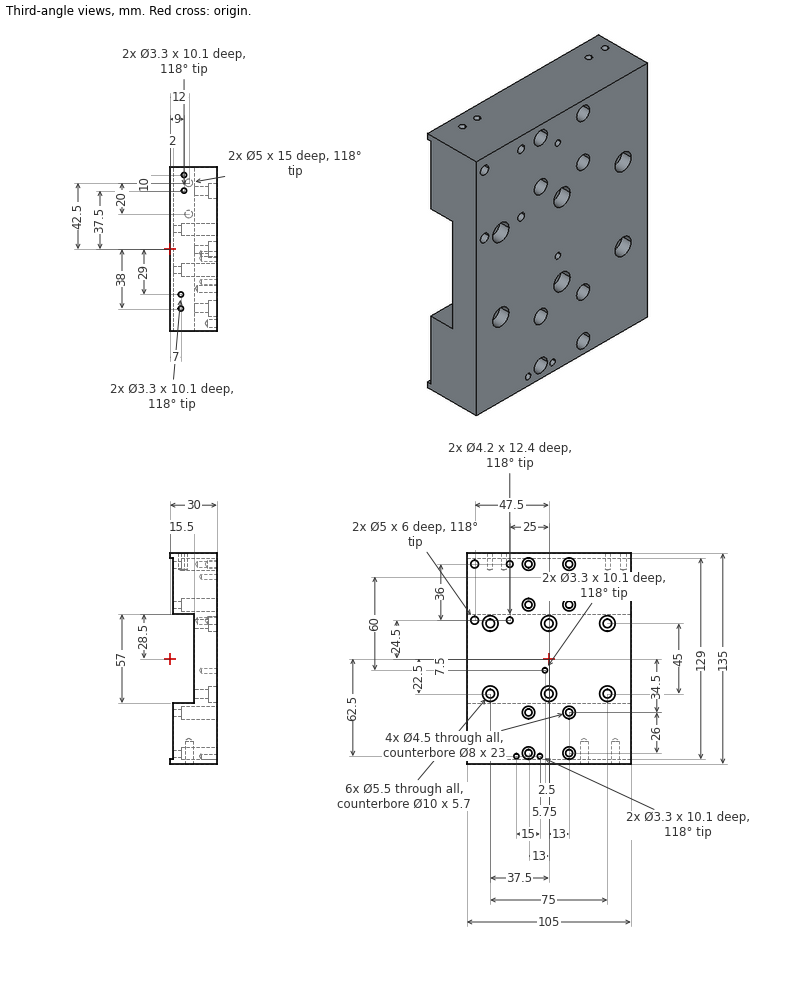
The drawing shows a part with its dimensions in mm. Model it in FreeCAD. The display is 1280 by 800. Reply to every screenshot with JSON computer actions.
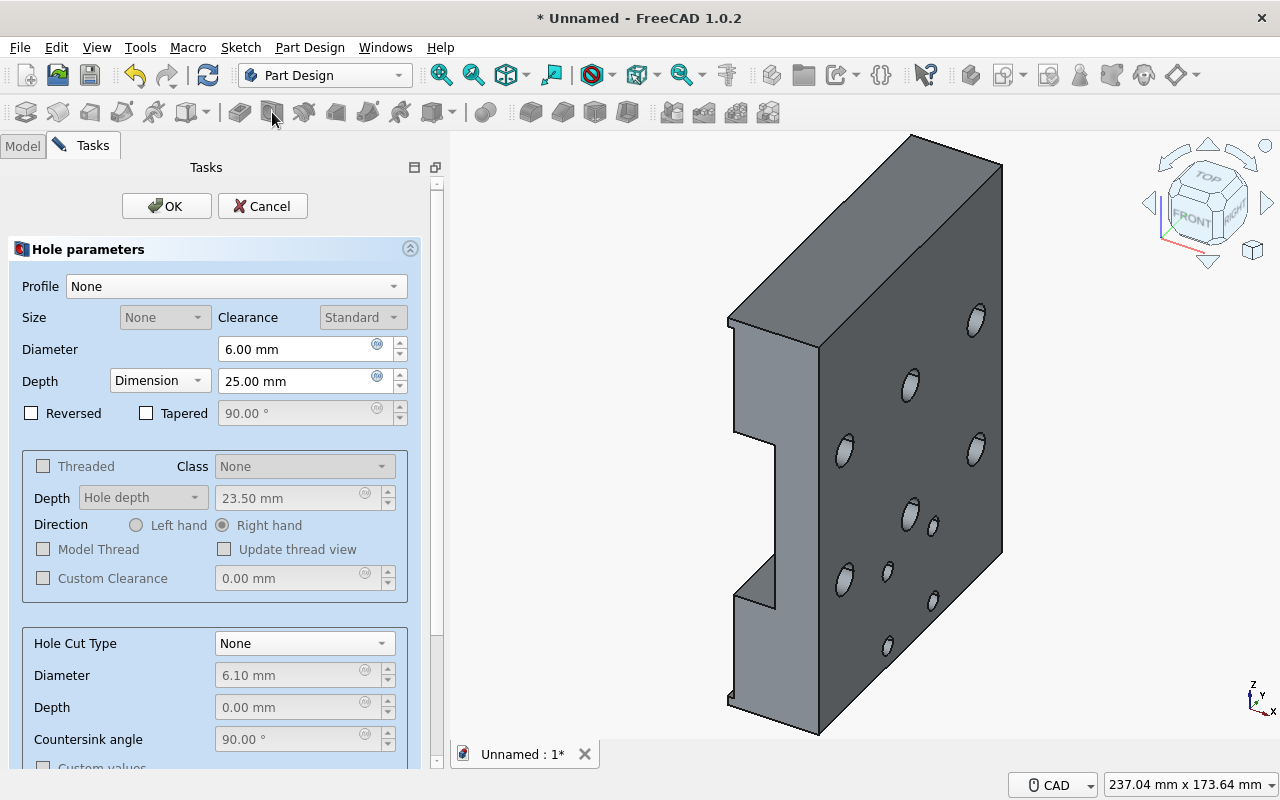
{"action": "triple_click", "coordinate": [305, 349]}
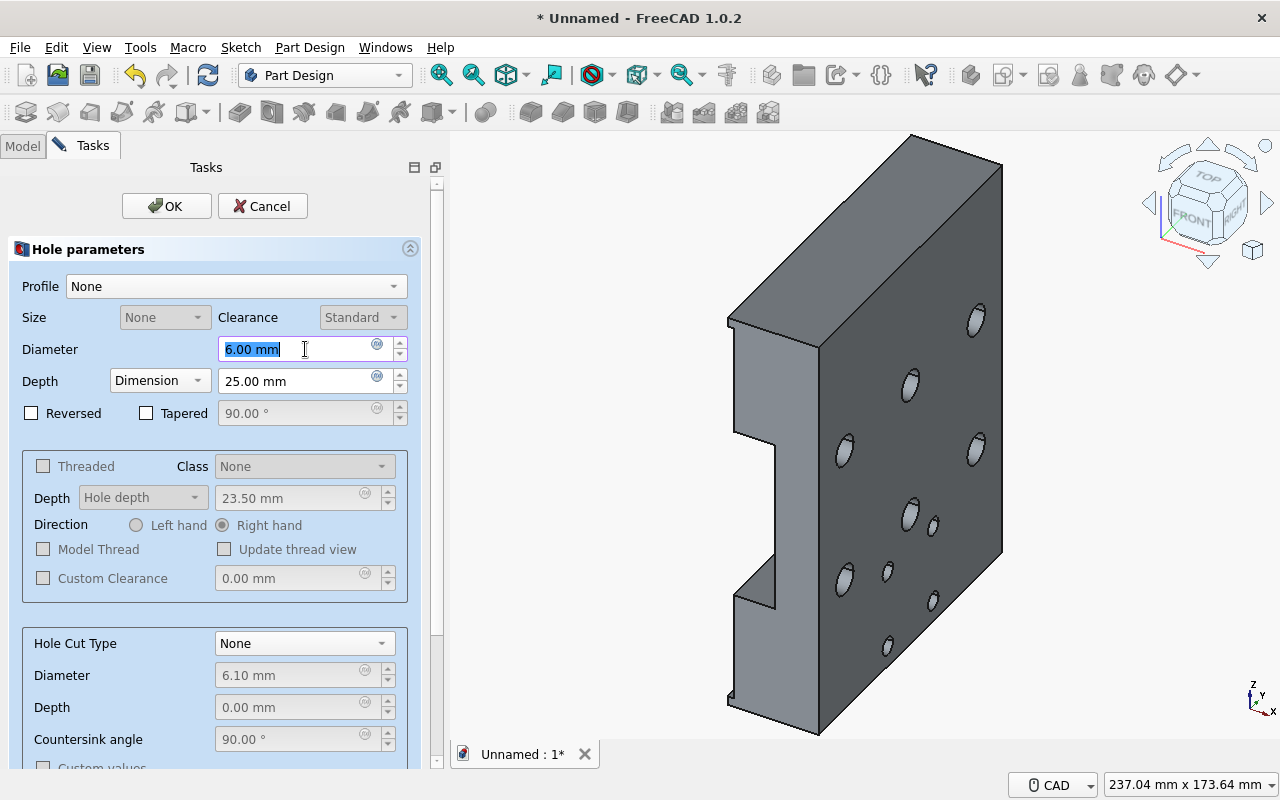
{"action": "type", "text": "4.5"}
{"action": "key", "text": "Tab"}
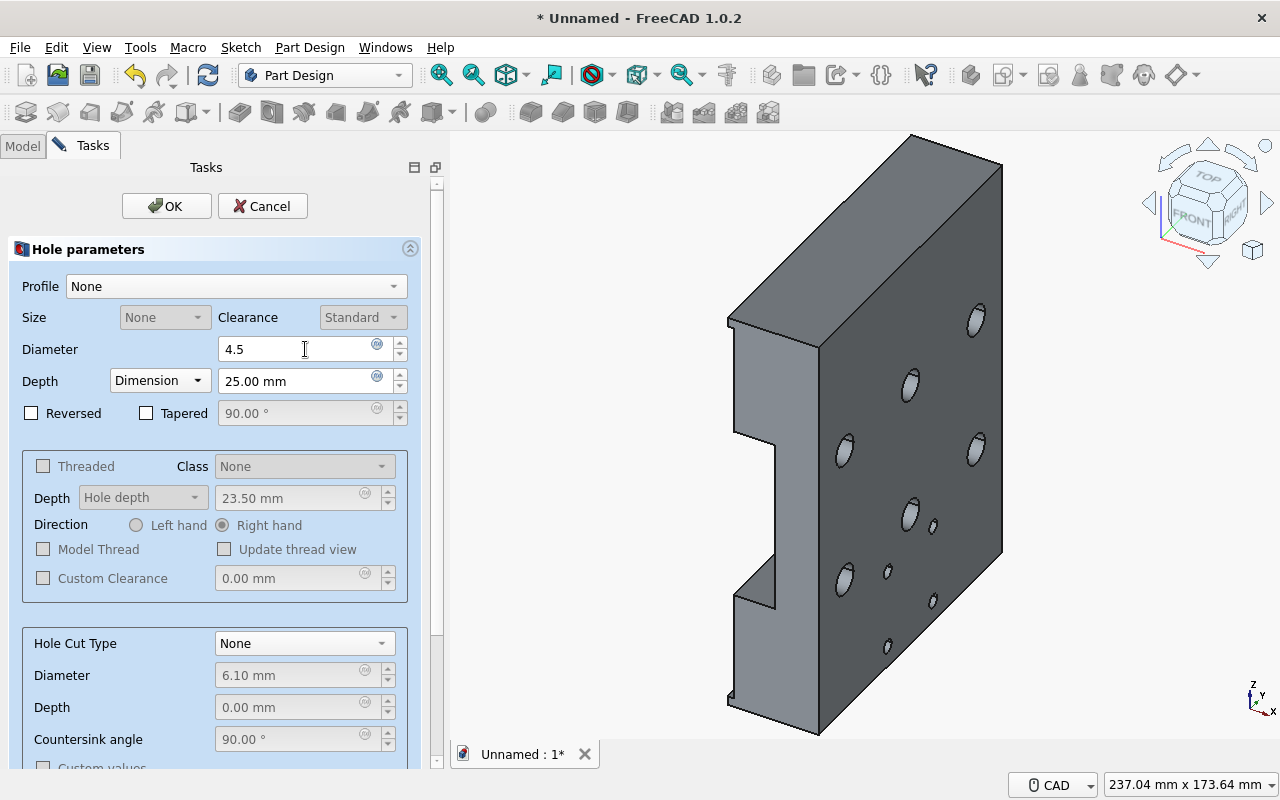
{"action": "left_click", "coordinate": [161, 380]}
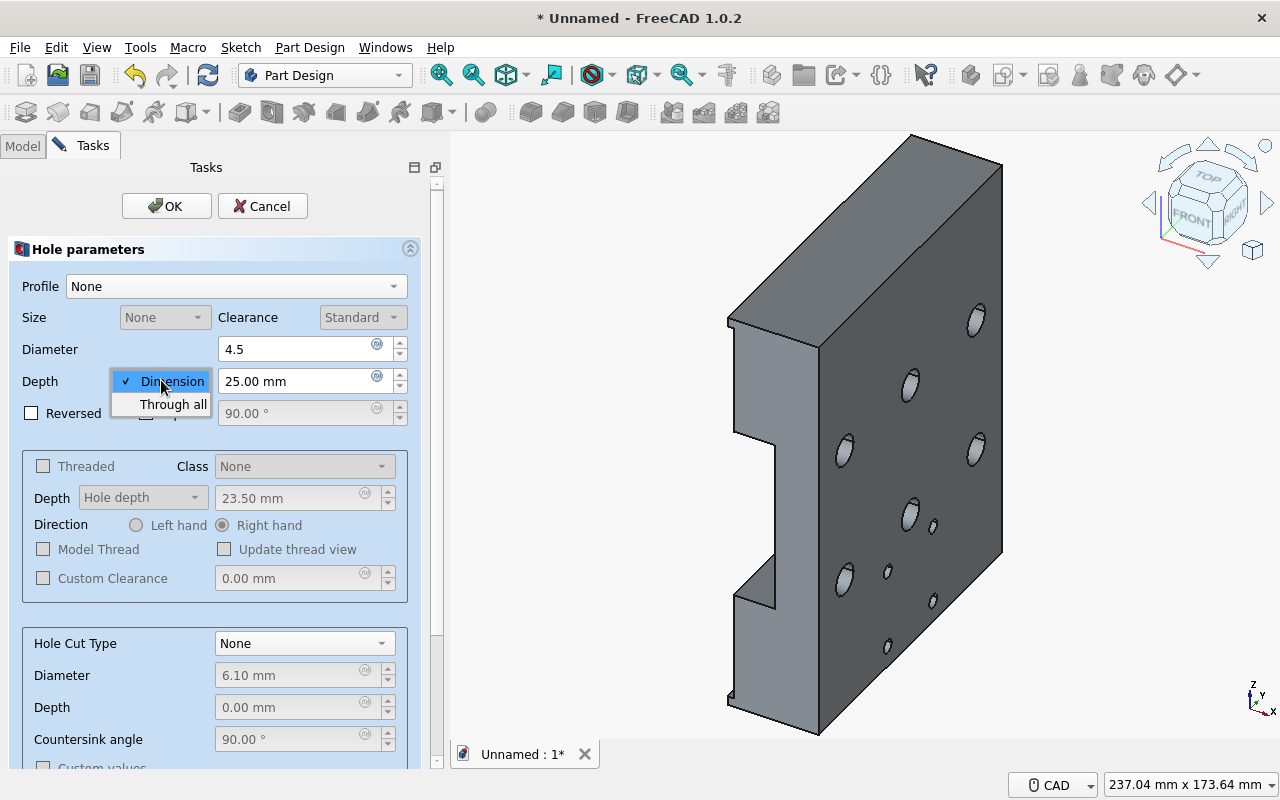
{"action": "left_click", "coordinate": [160, 404]}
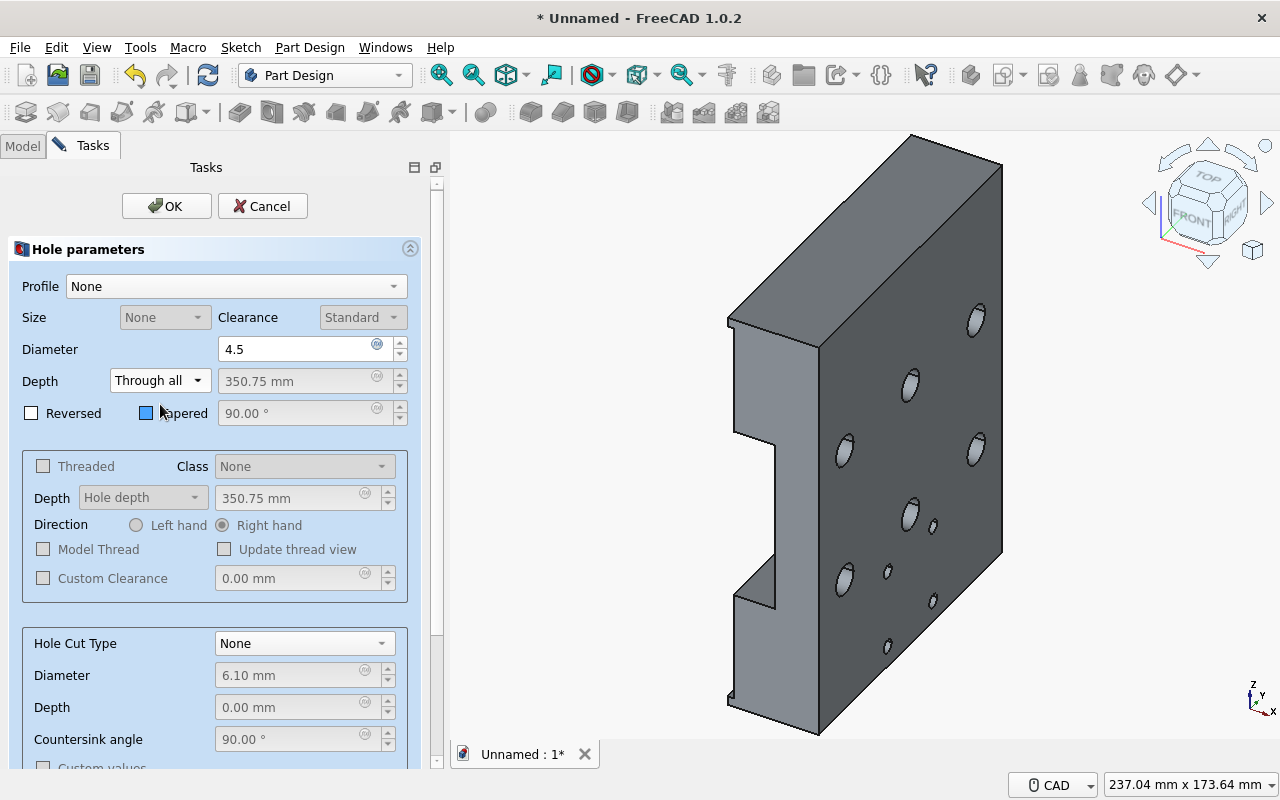
{"action": "left_click", "coordinate": [306, 644]}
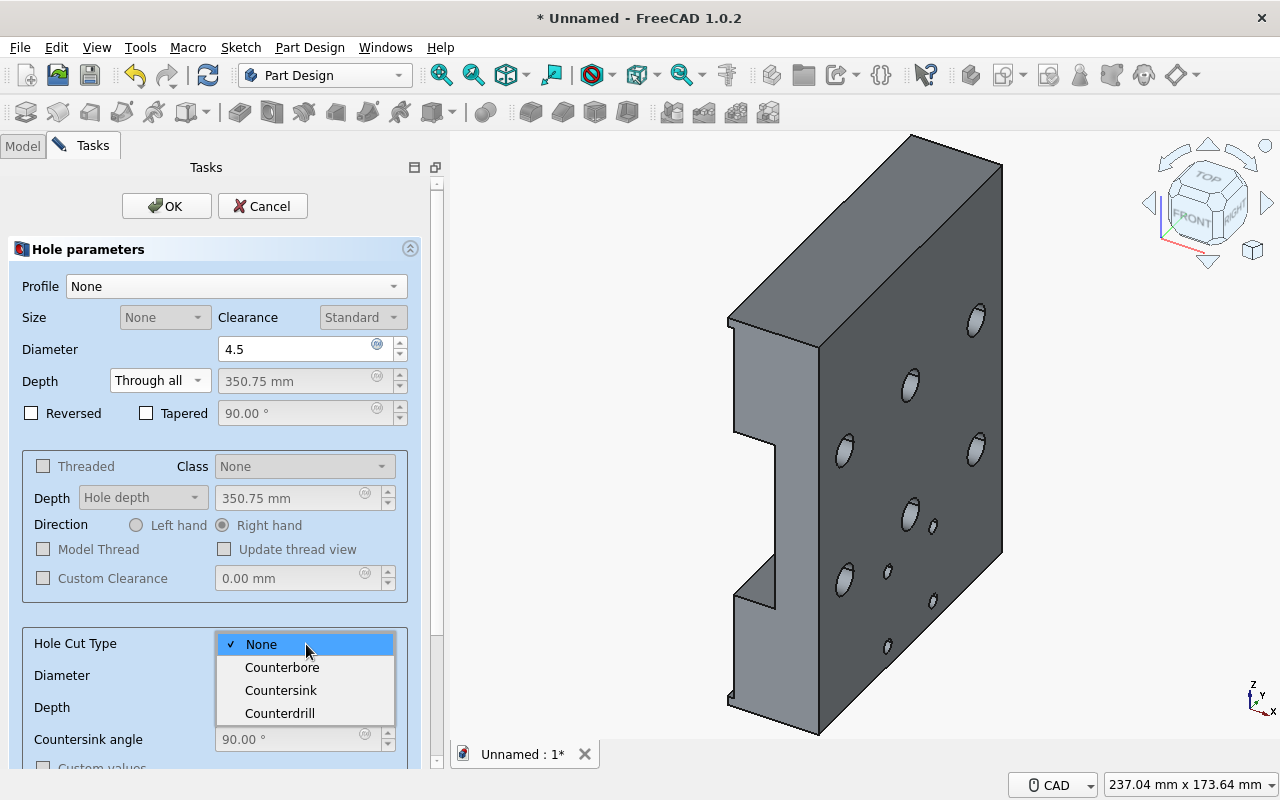
{"action": "left_click", "coordinate": [304, 668]}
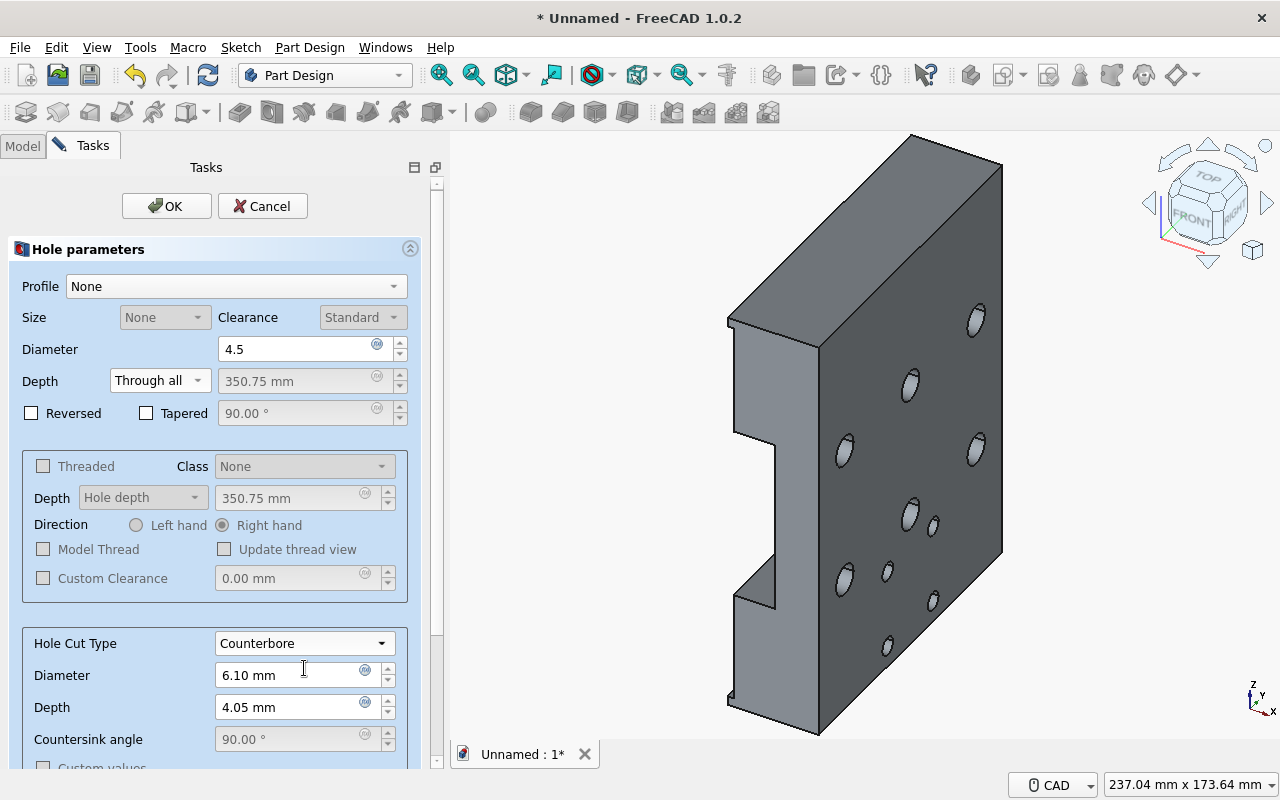
{"action": "triple_click", "coordinate": [298, 675]}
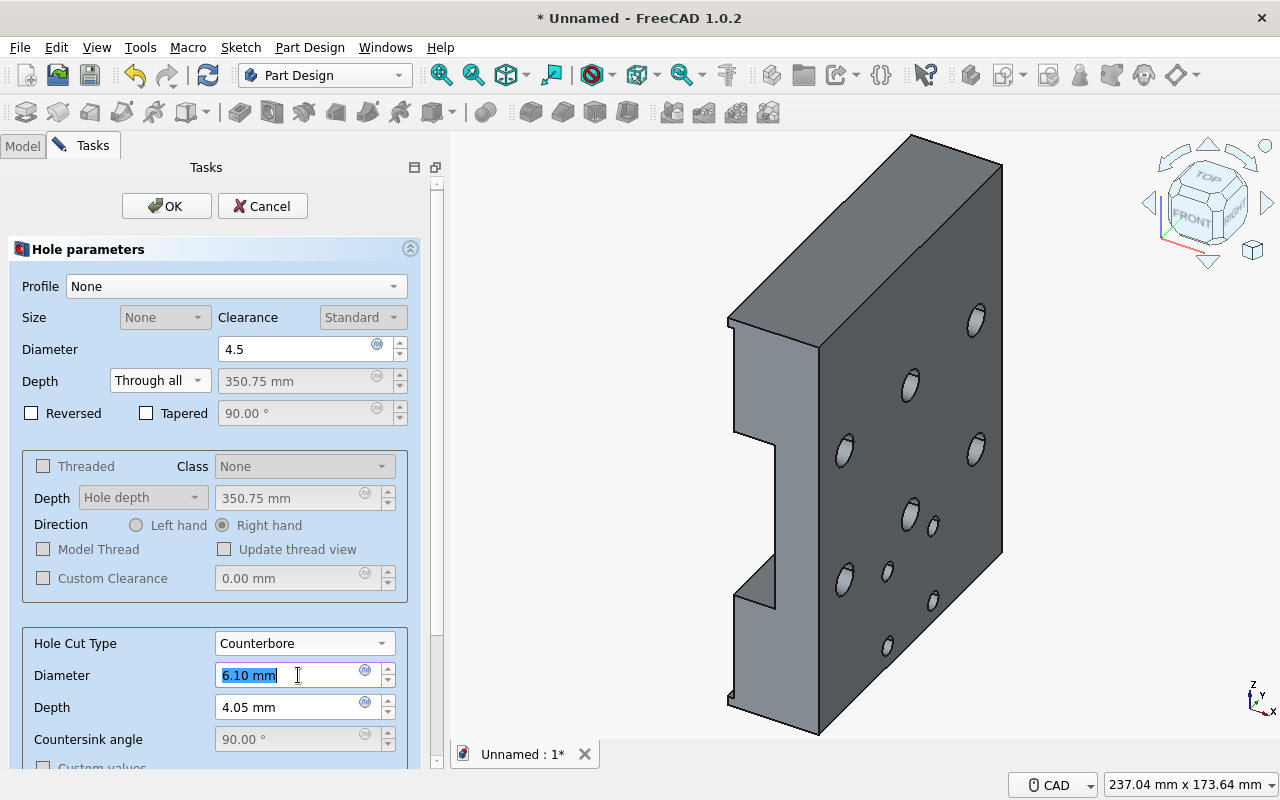
{"action": "type", "text": "8"}
{"action": "key", "text": "Tab"}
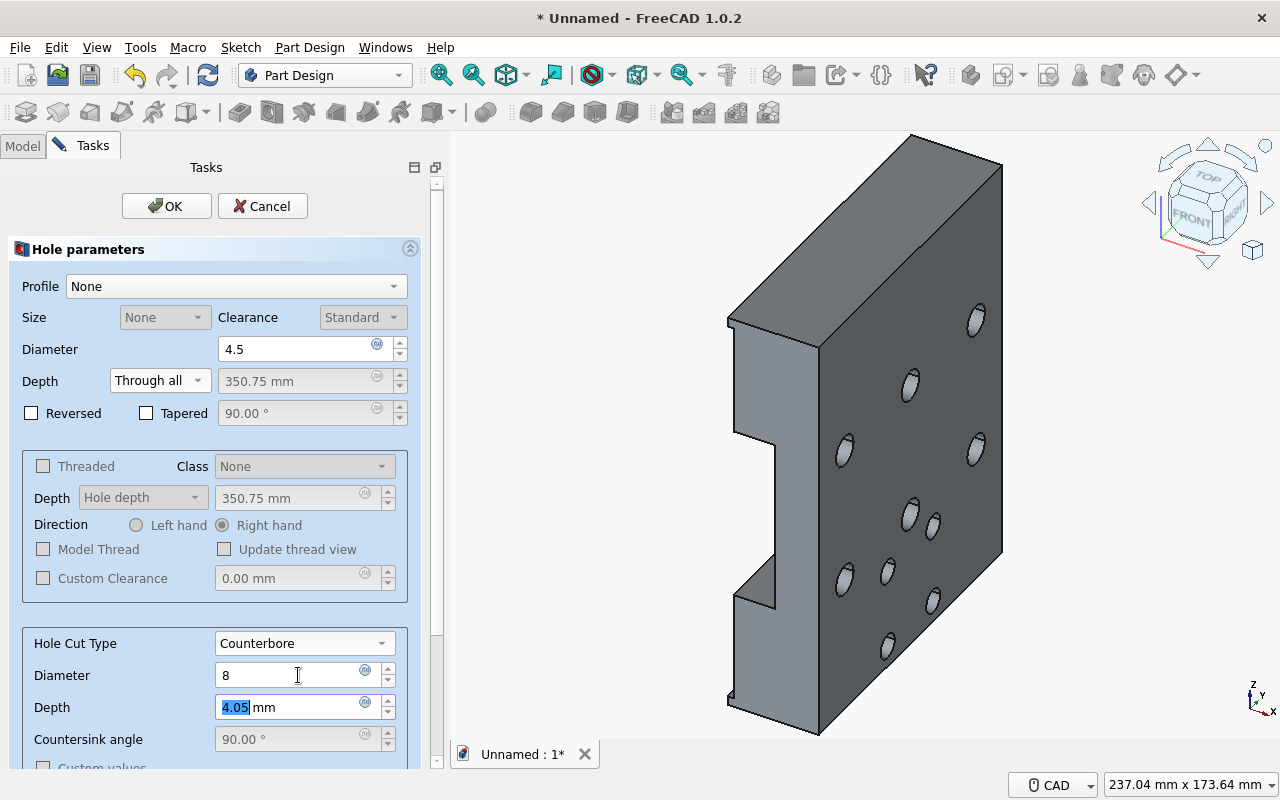
{"action": "type", "text": "23"}
{"action": "key", "text": "Tab"}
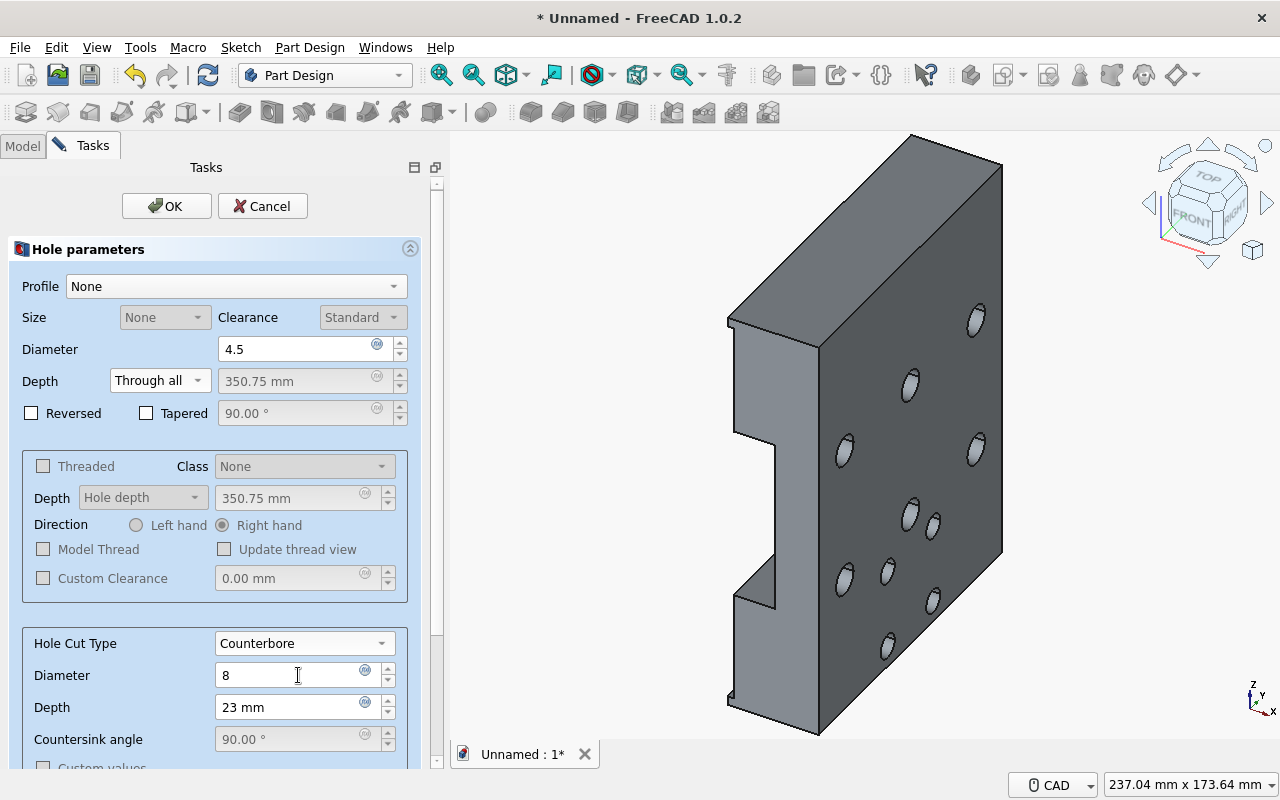
{"action": "left_click", "coordinate": [167, 206]}